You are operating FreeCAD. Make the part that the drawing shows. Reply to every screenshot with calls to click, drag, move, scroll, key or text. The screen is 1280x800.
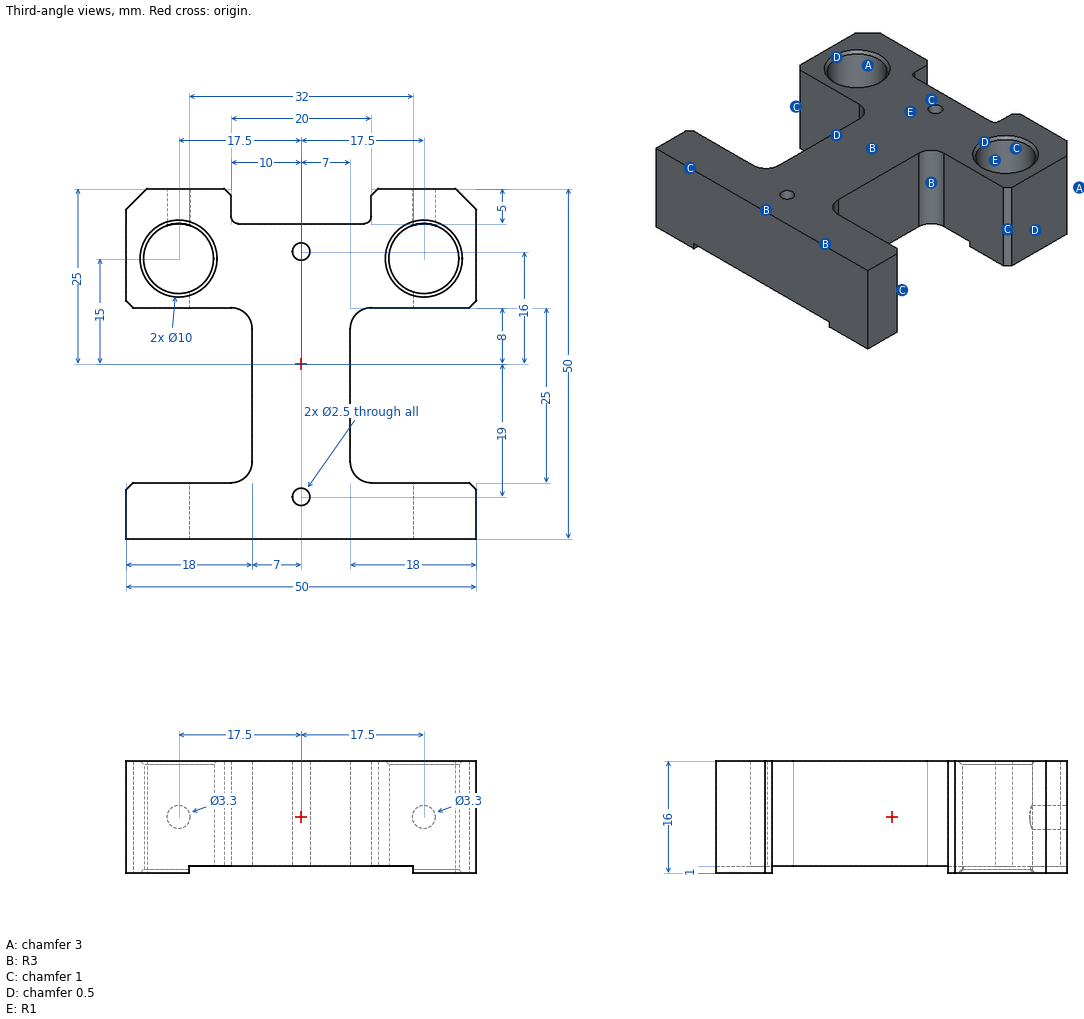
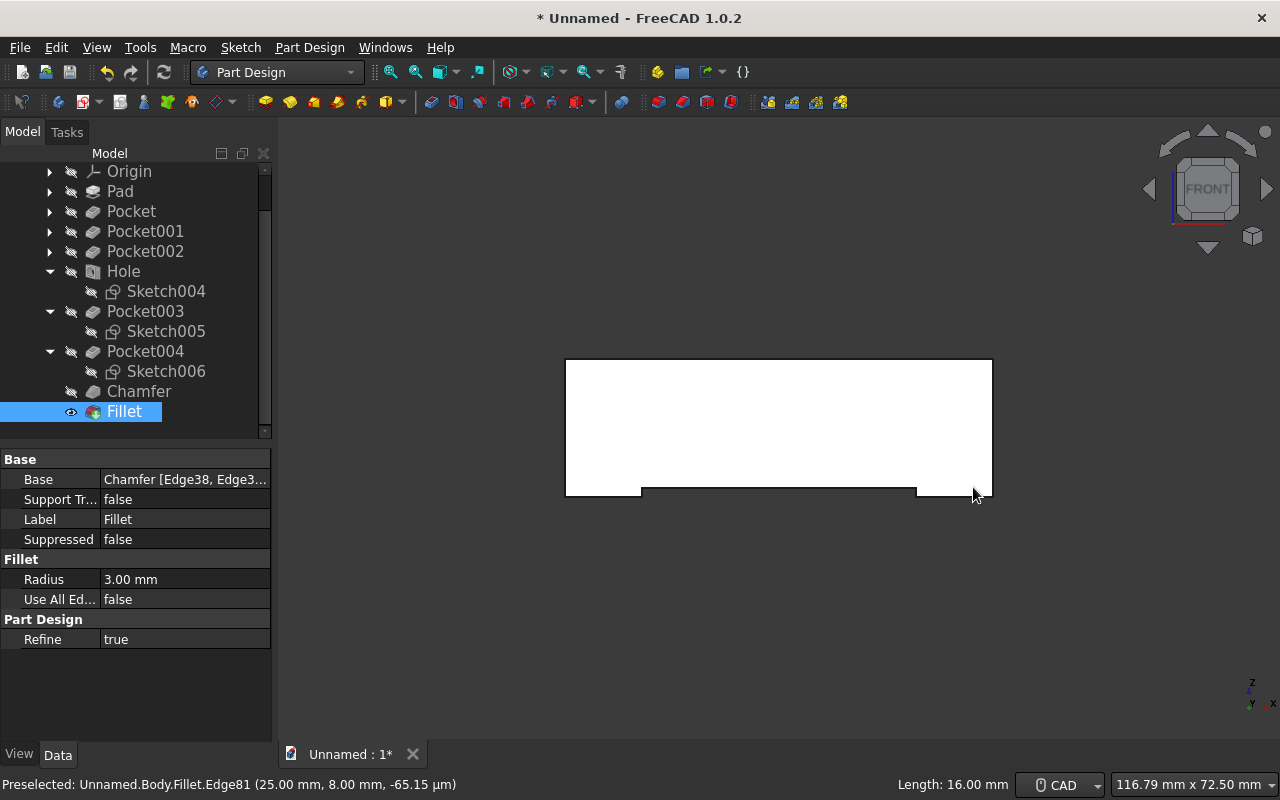
click(392, 72)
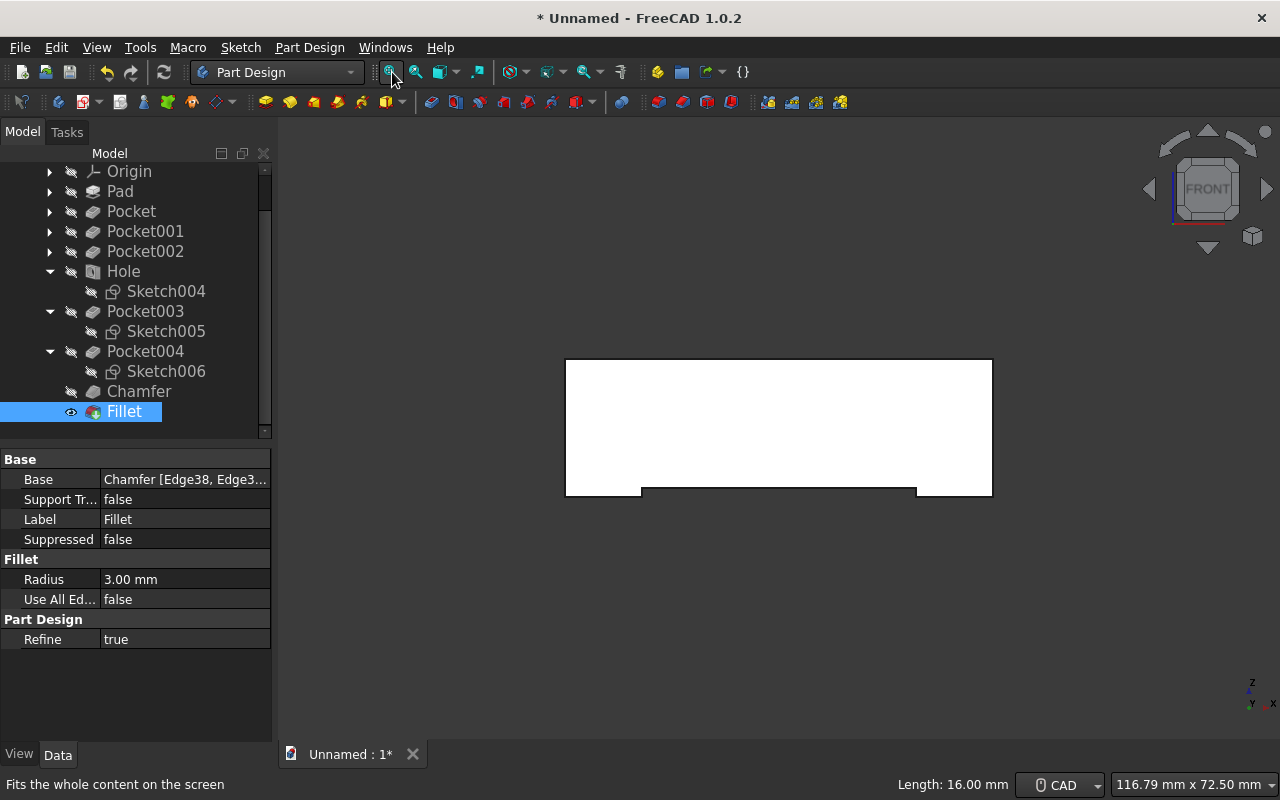
key(3)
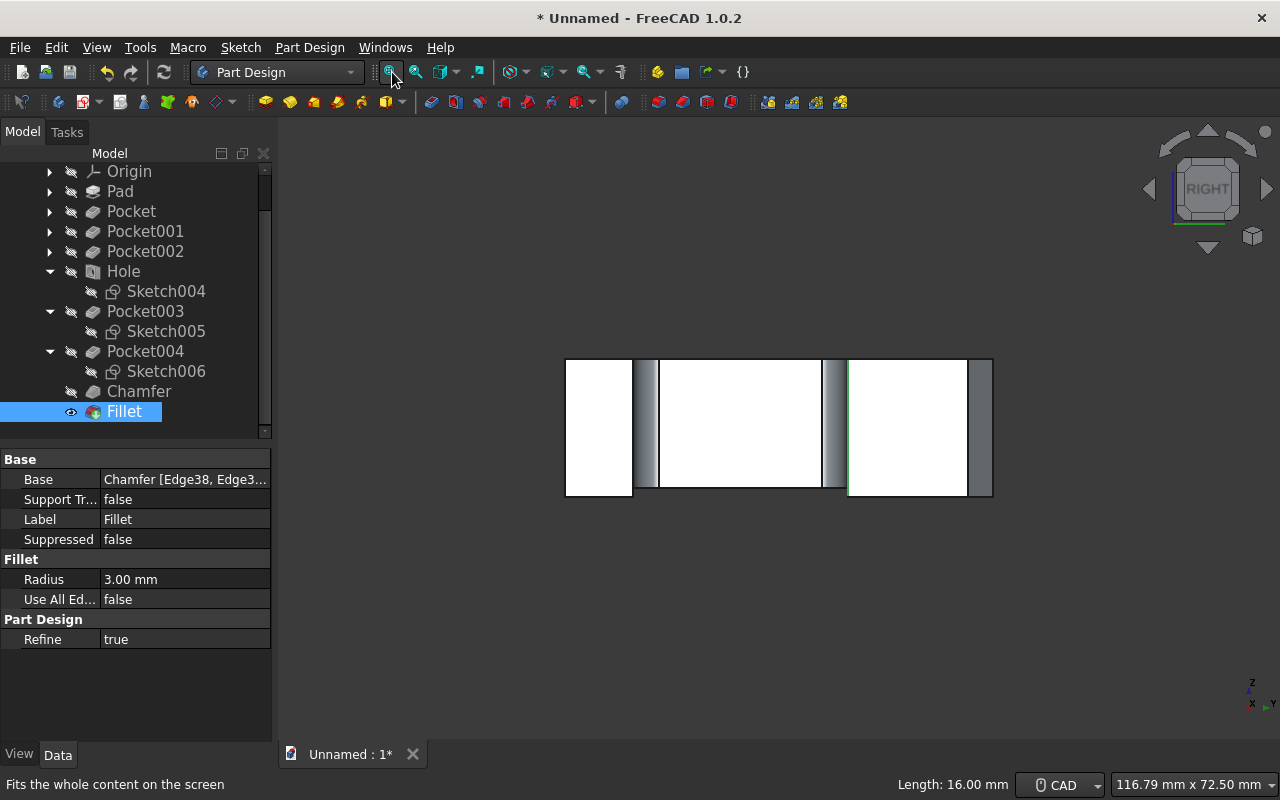
key(v)
key(f)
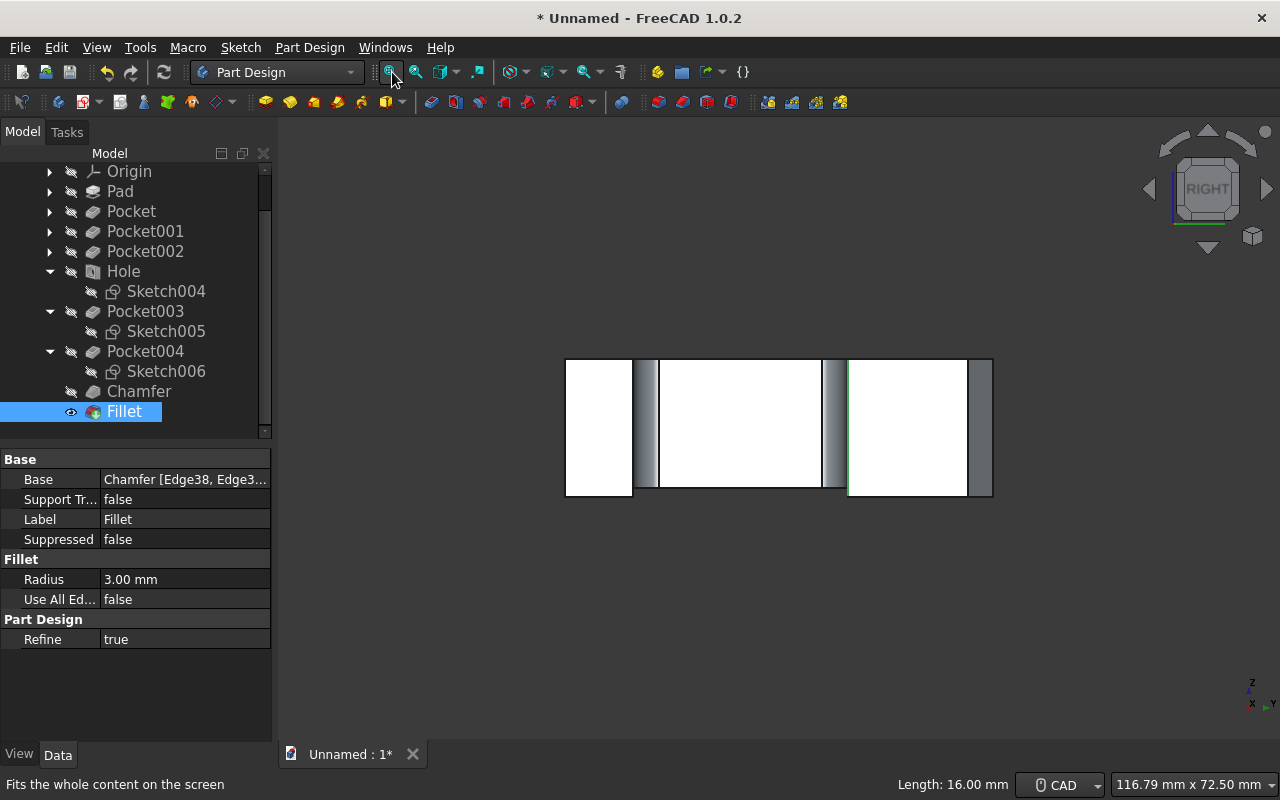
click(633, 427, ctrl)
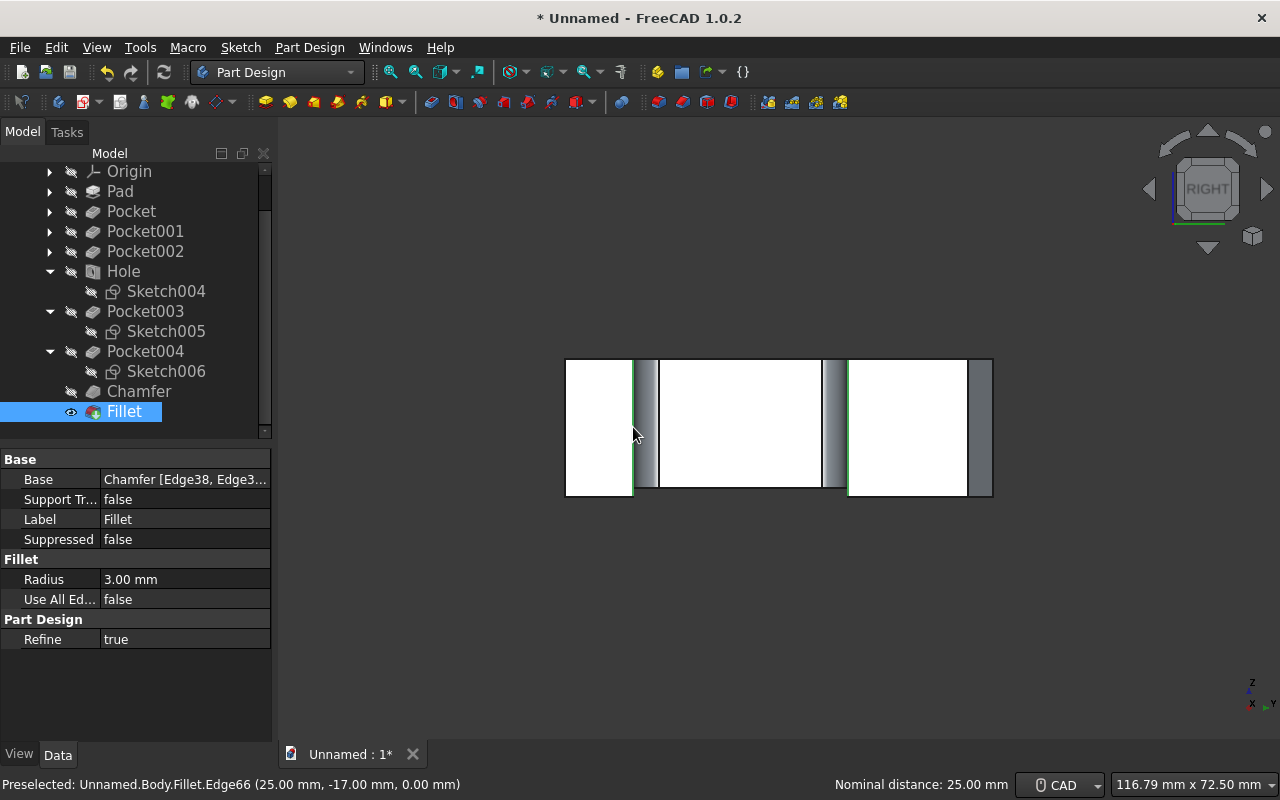
key(5)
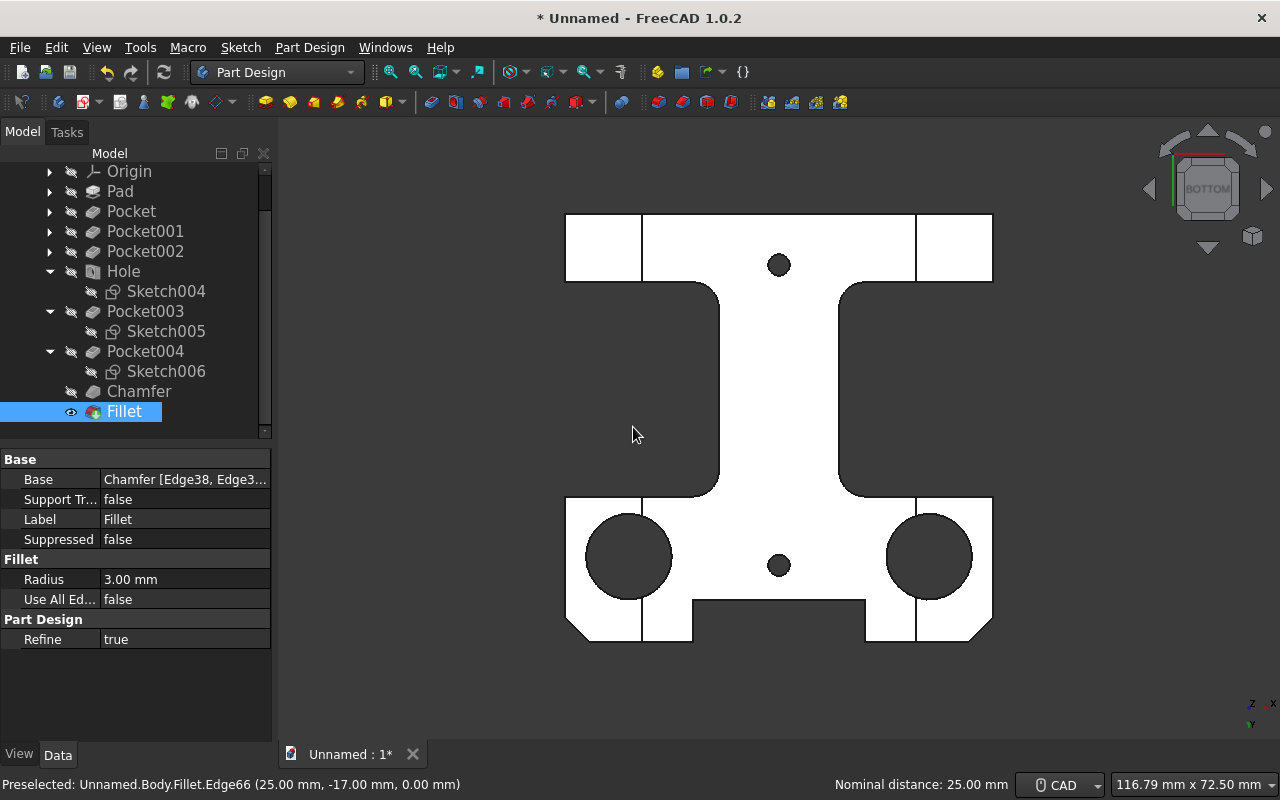
key(4)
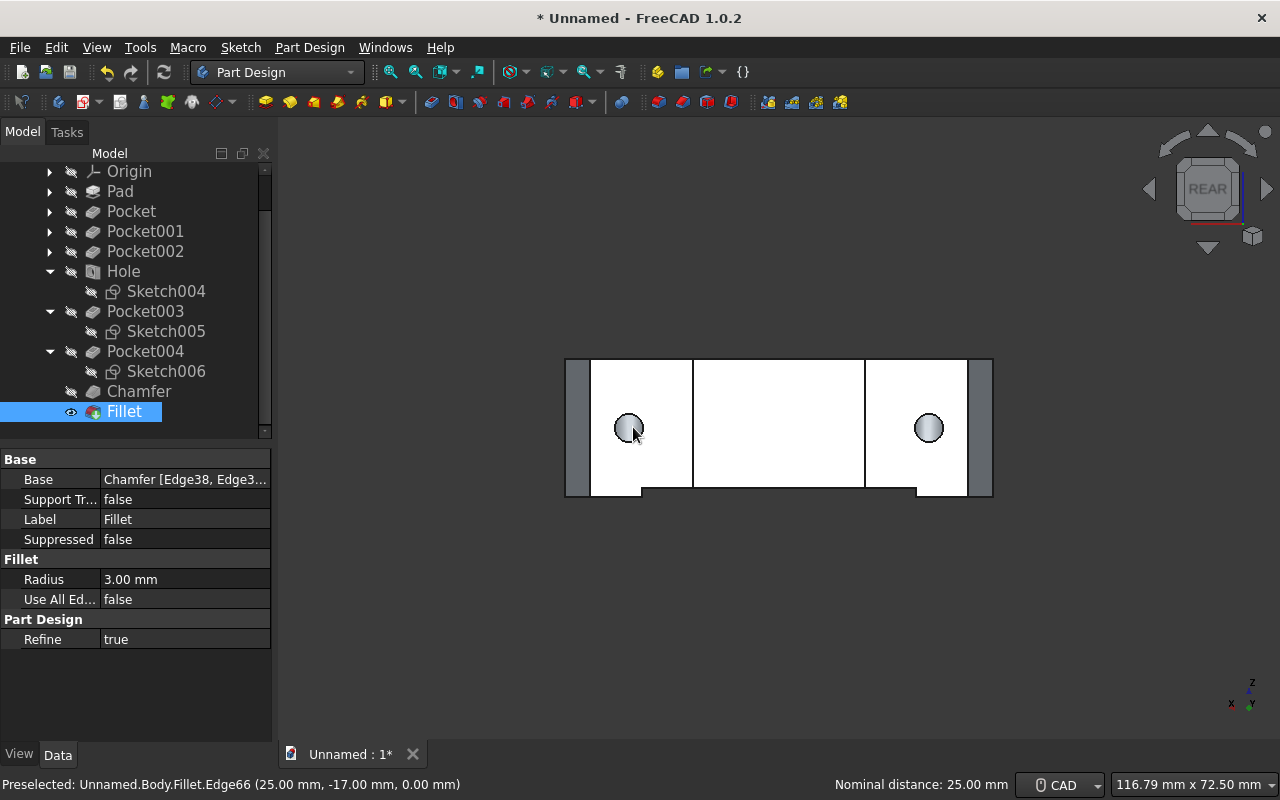
key(v)
key(f)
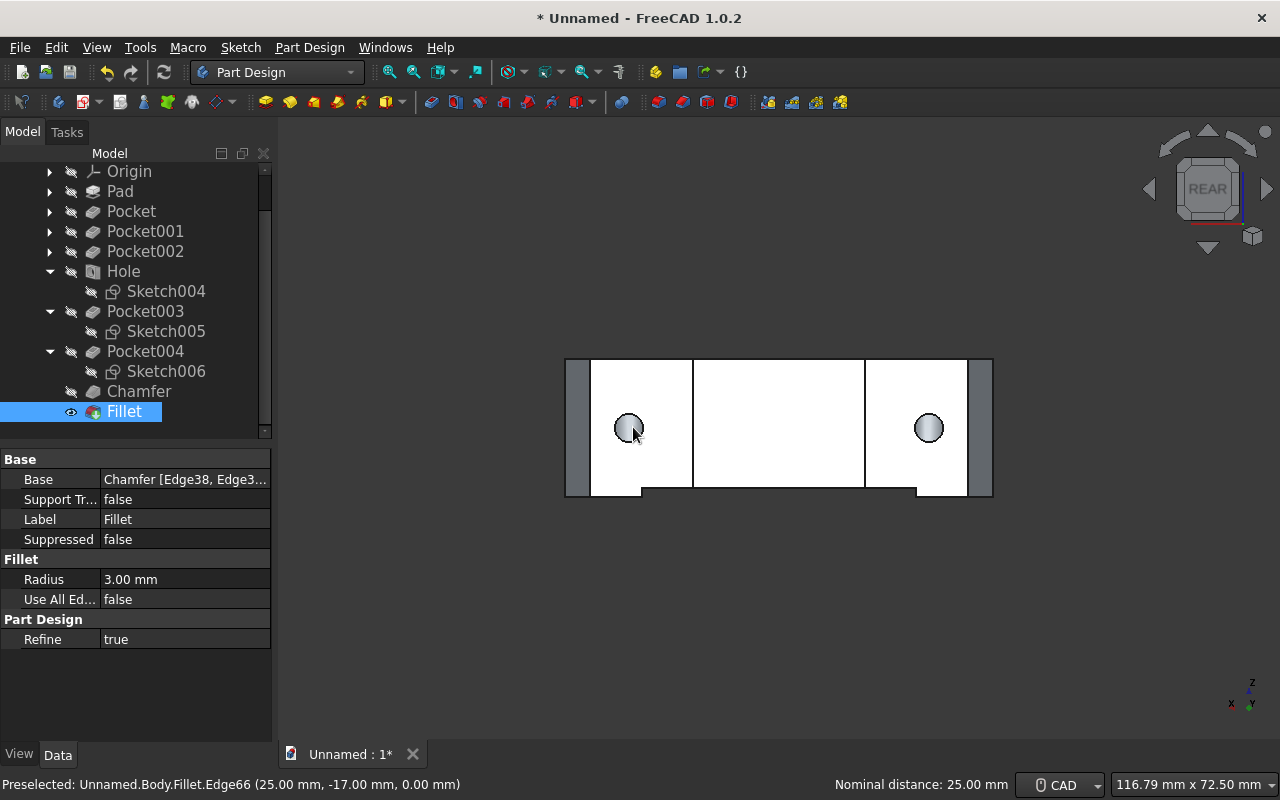
click(865, 423, ctrl)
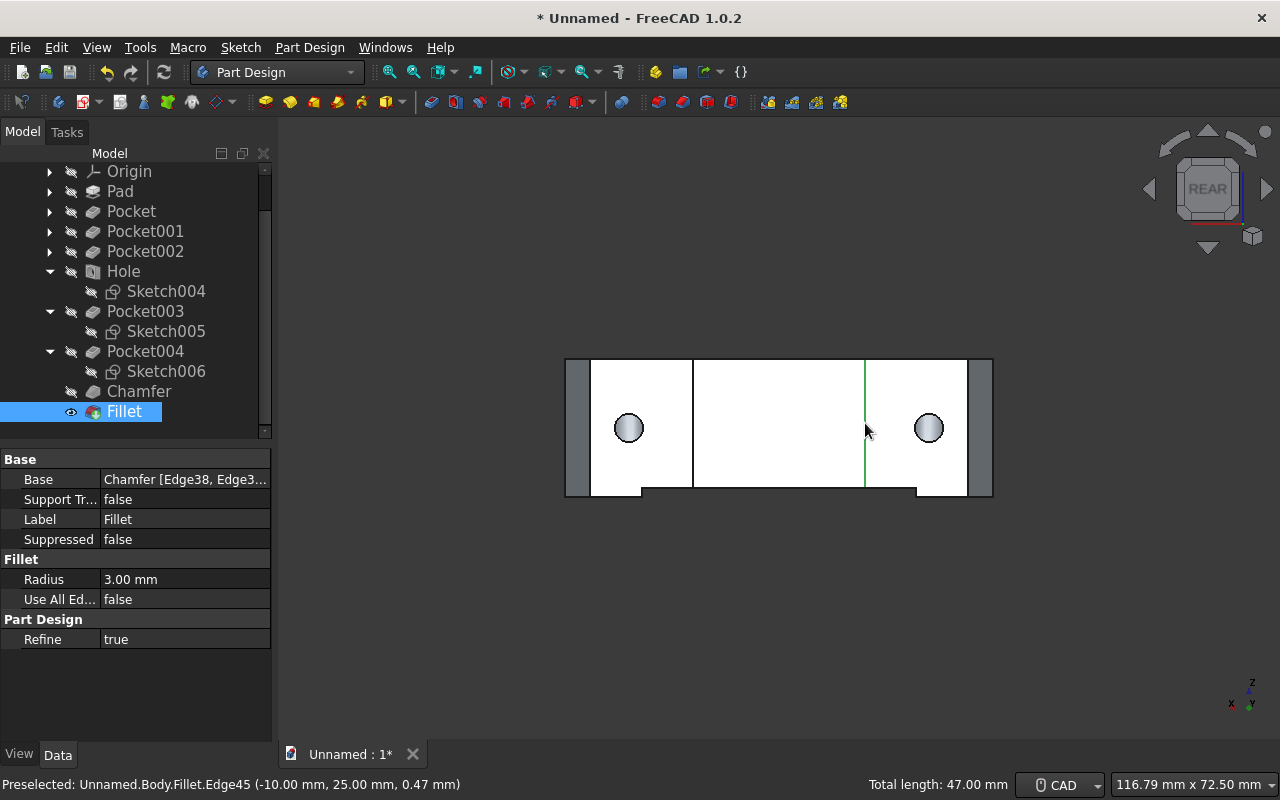
click(693, 423, ctrl)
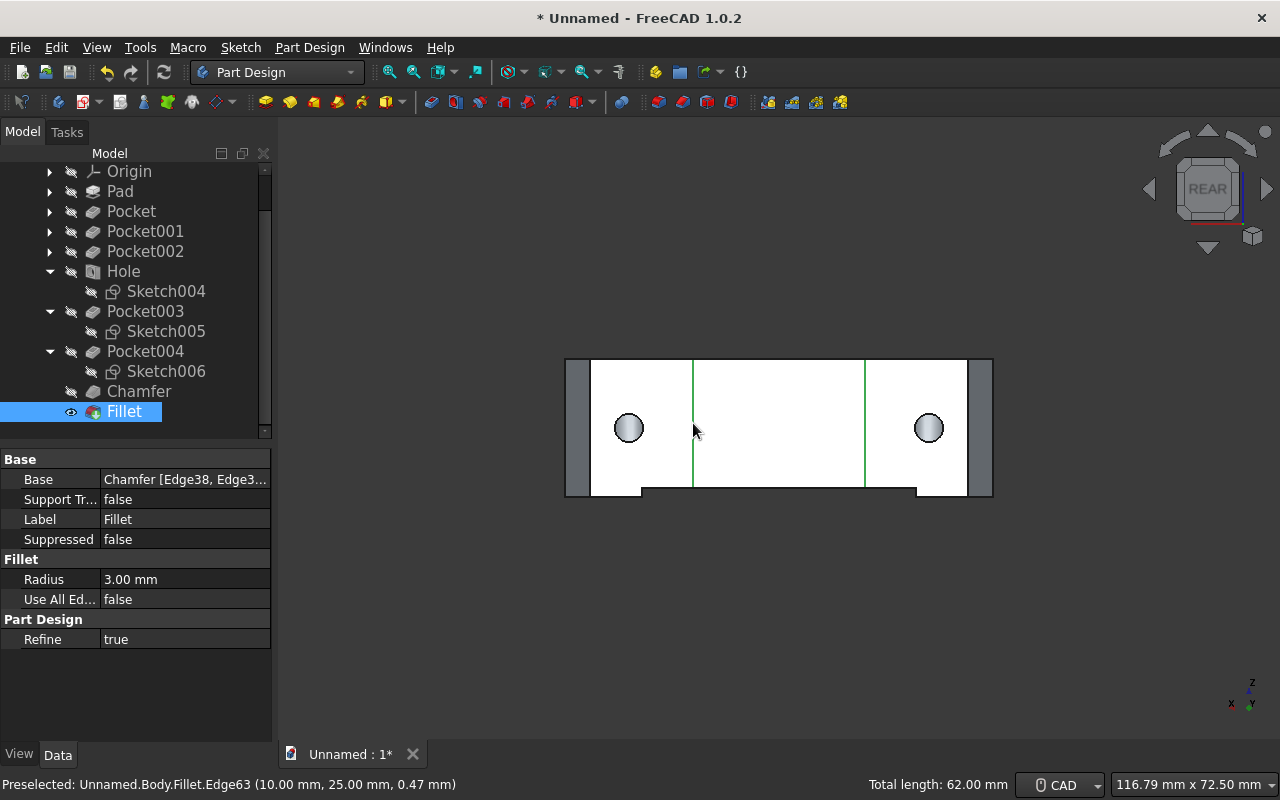
key(6)